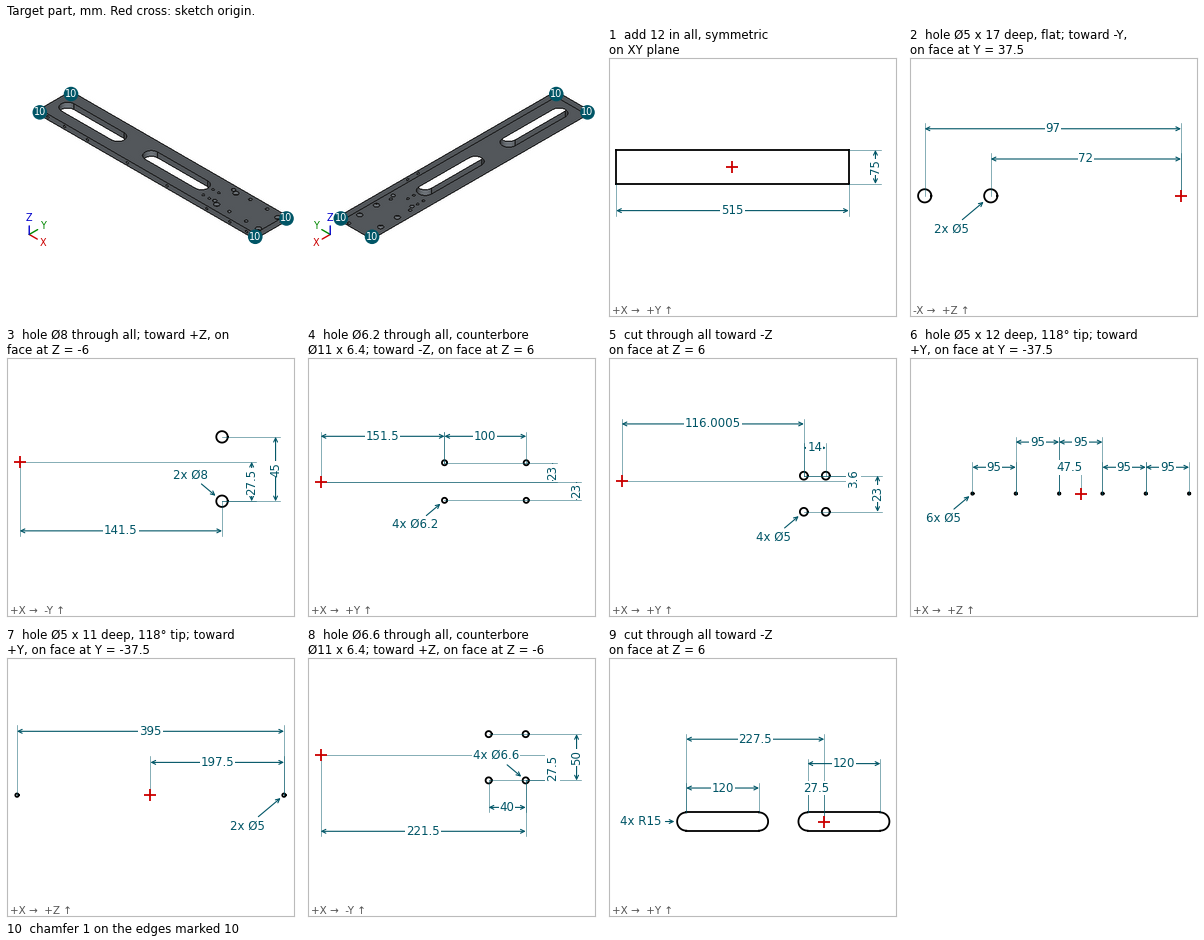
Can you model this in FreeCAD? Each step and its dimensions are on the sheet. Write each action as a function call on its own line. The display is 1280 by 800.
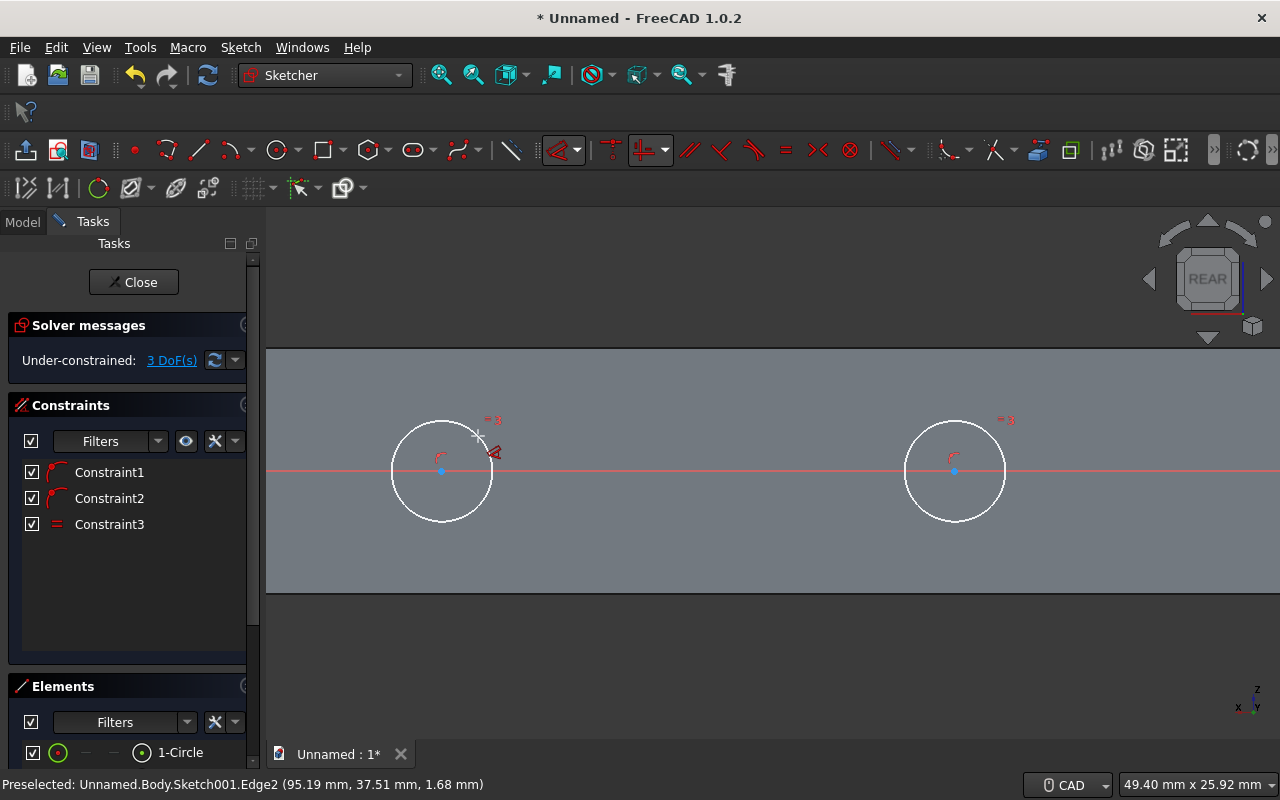
click(991, 436)
click(1014, 414)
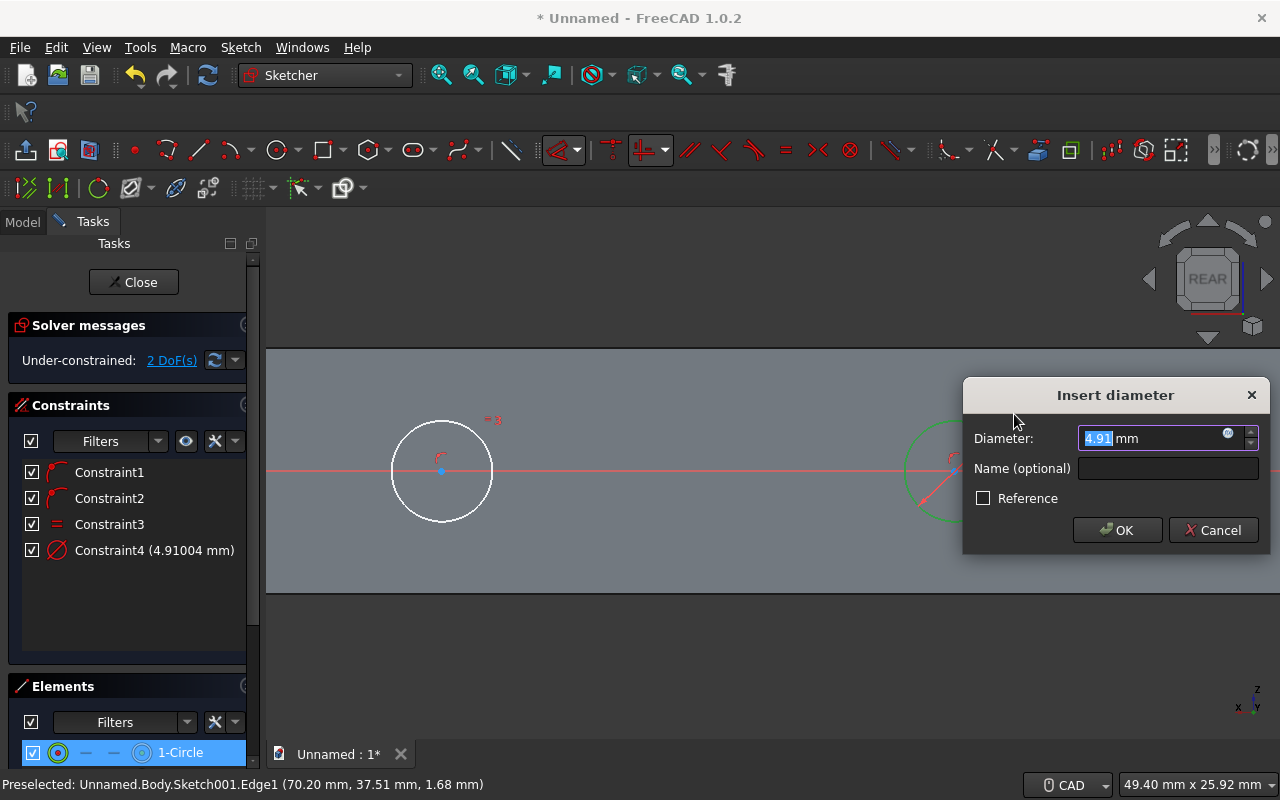
text(5)
key(Return)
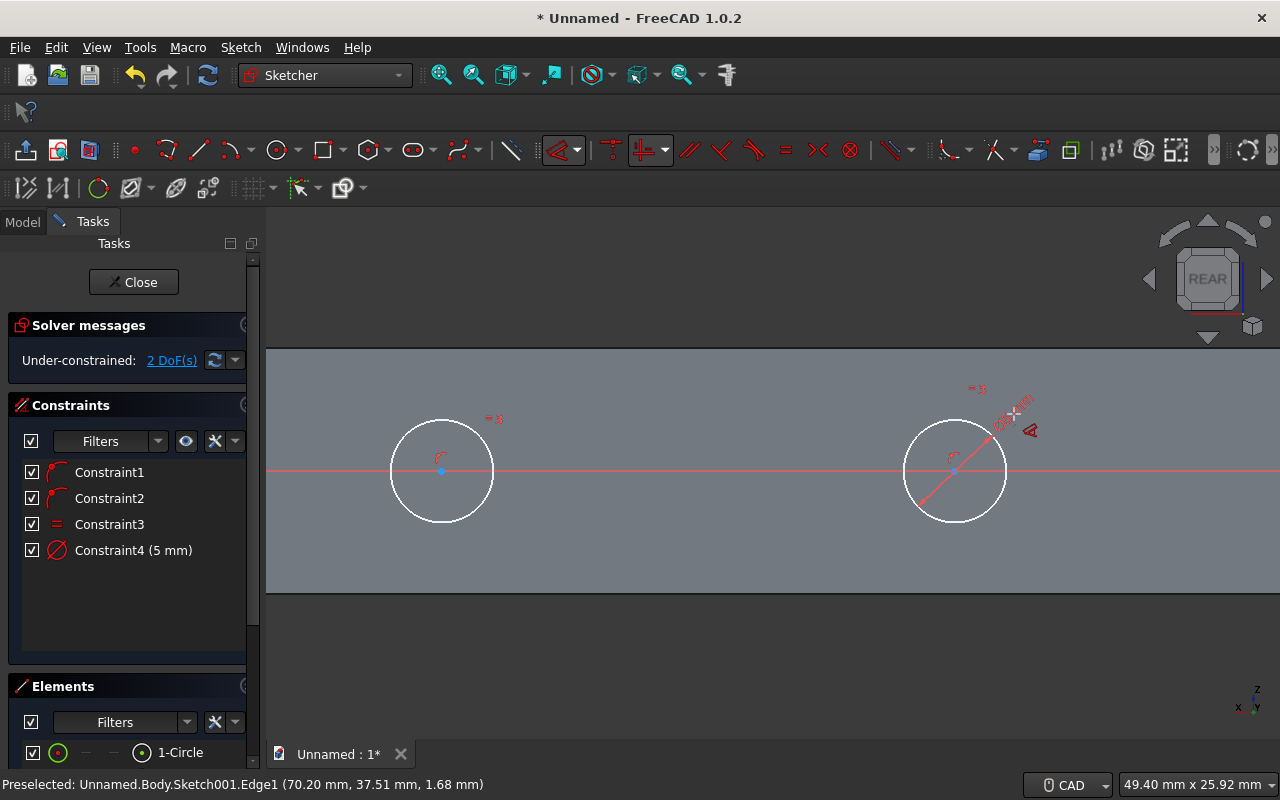
click(955, 471)
click(1035, 505)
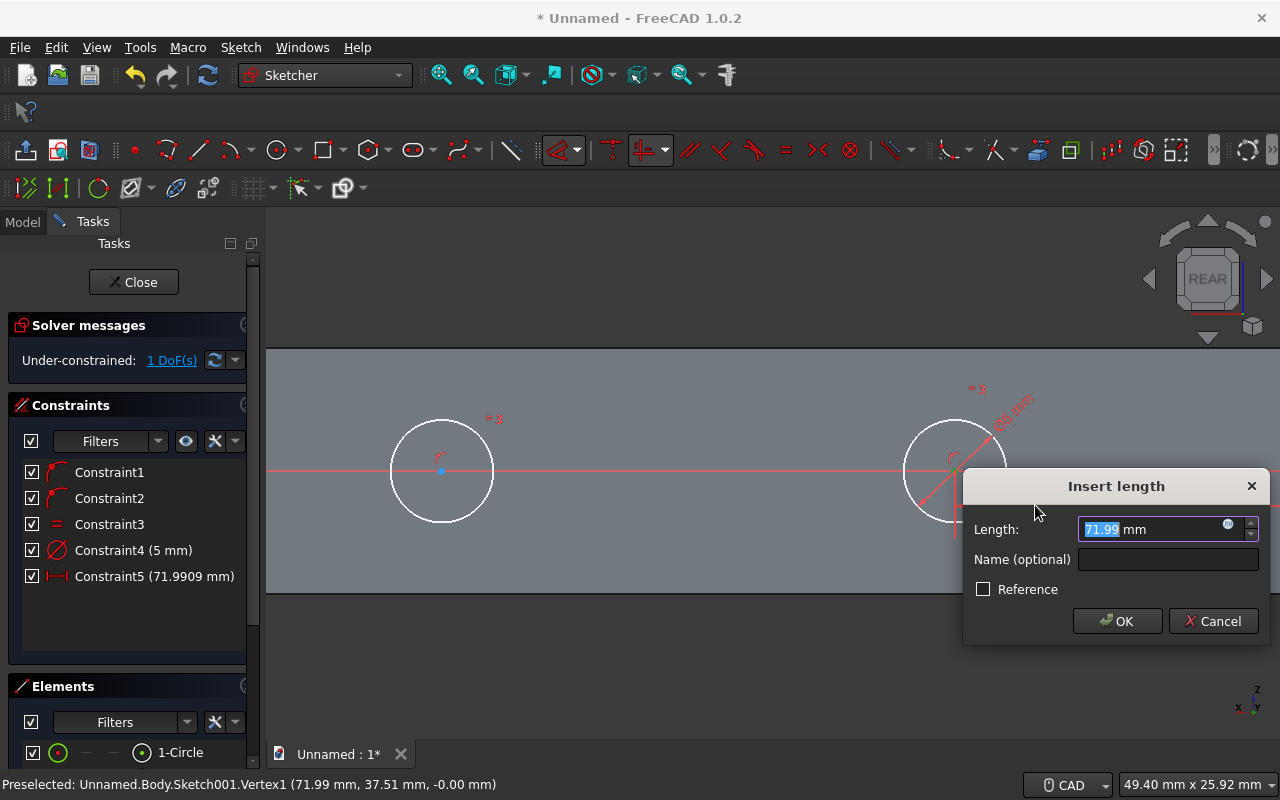
text(72)
key(Return)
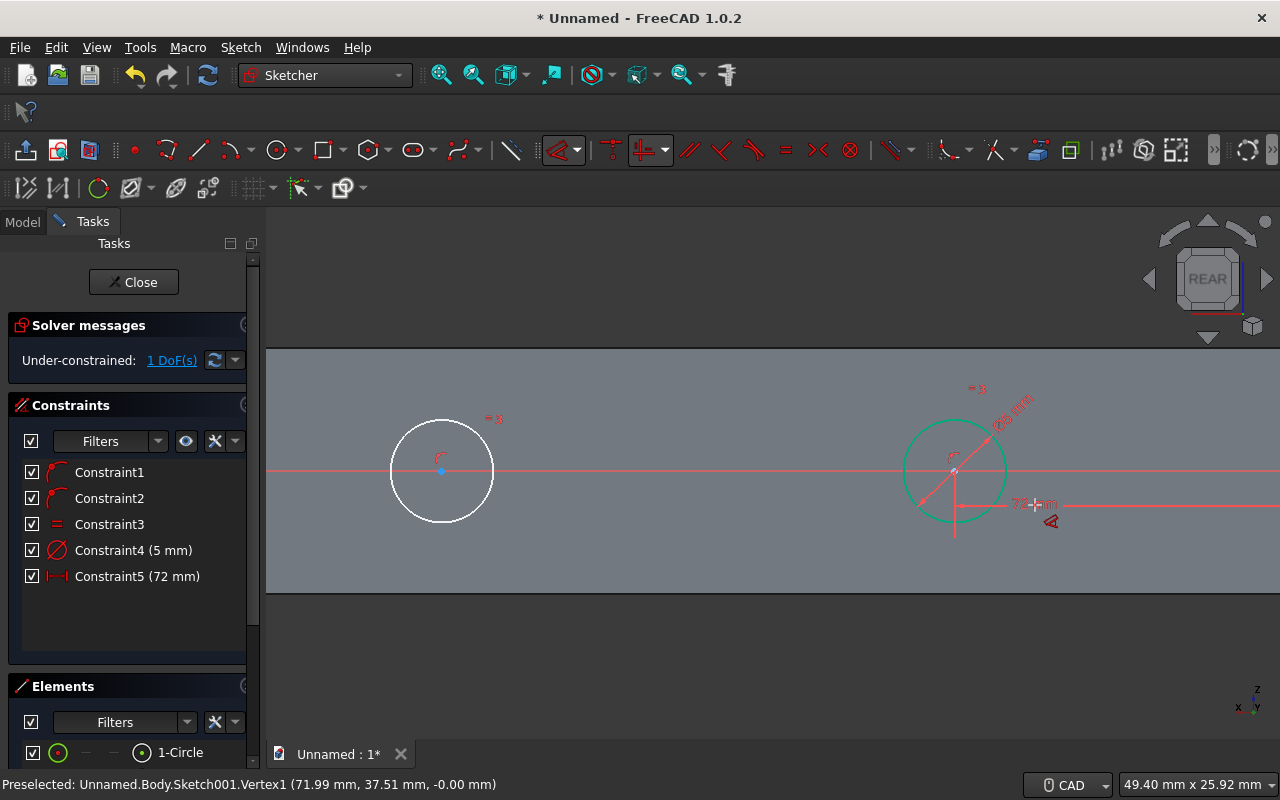
click(442, 471)
click(779, 505)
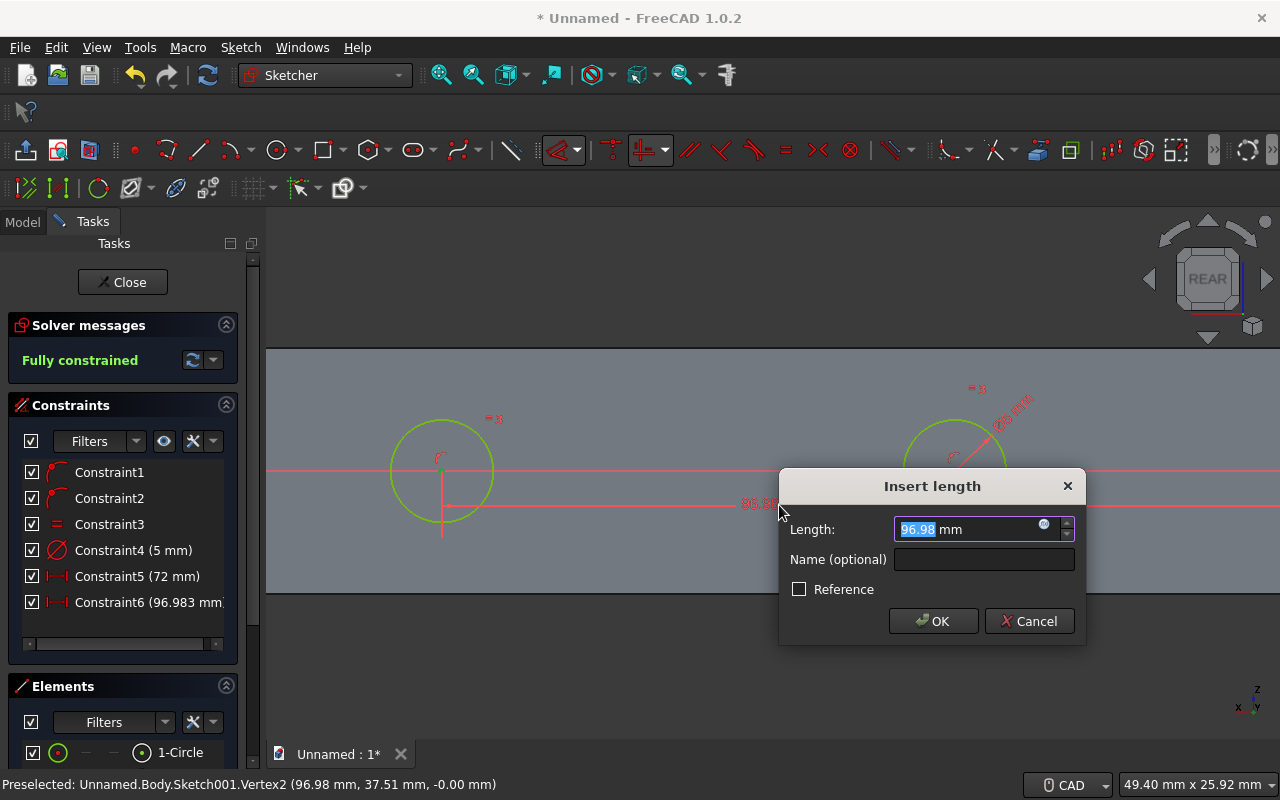
text(97)
key(Return)
key(Escape)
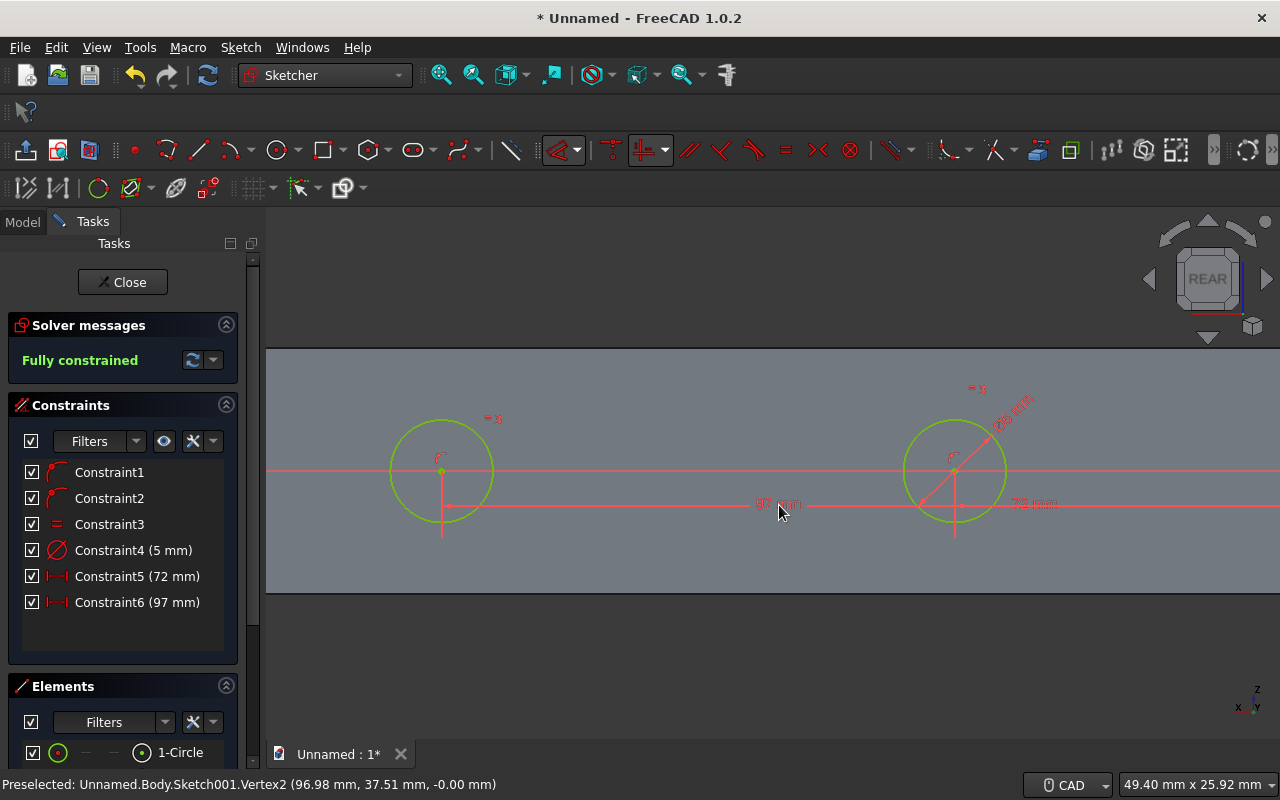
click(123, 282)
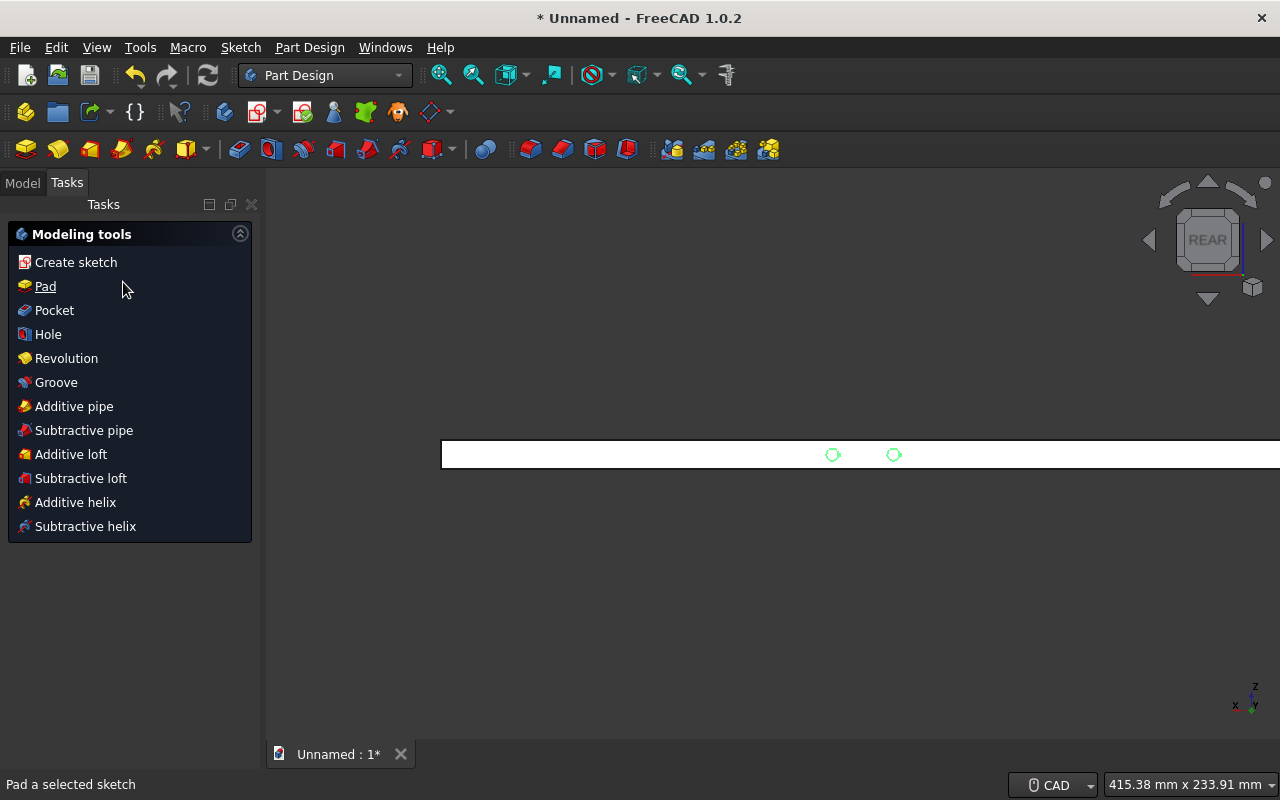
click(272, 150)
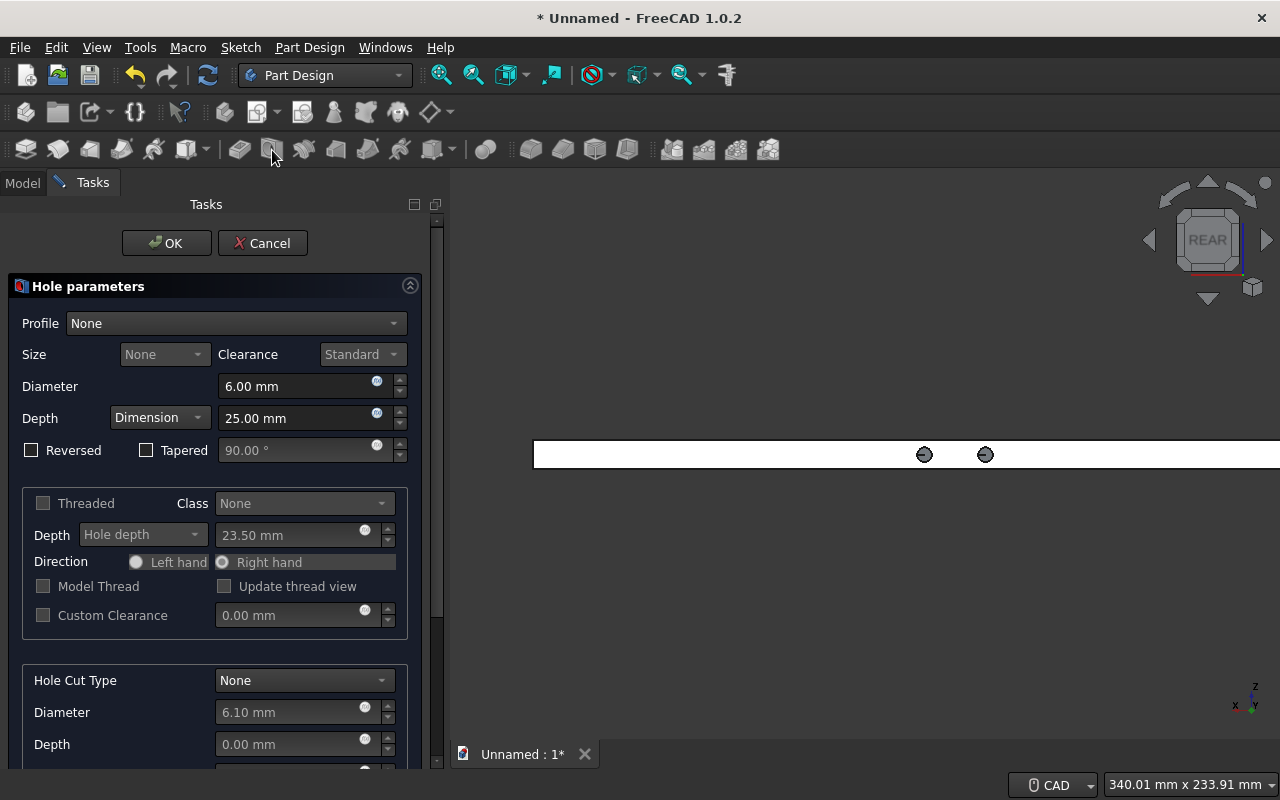
triple_click(305, 386)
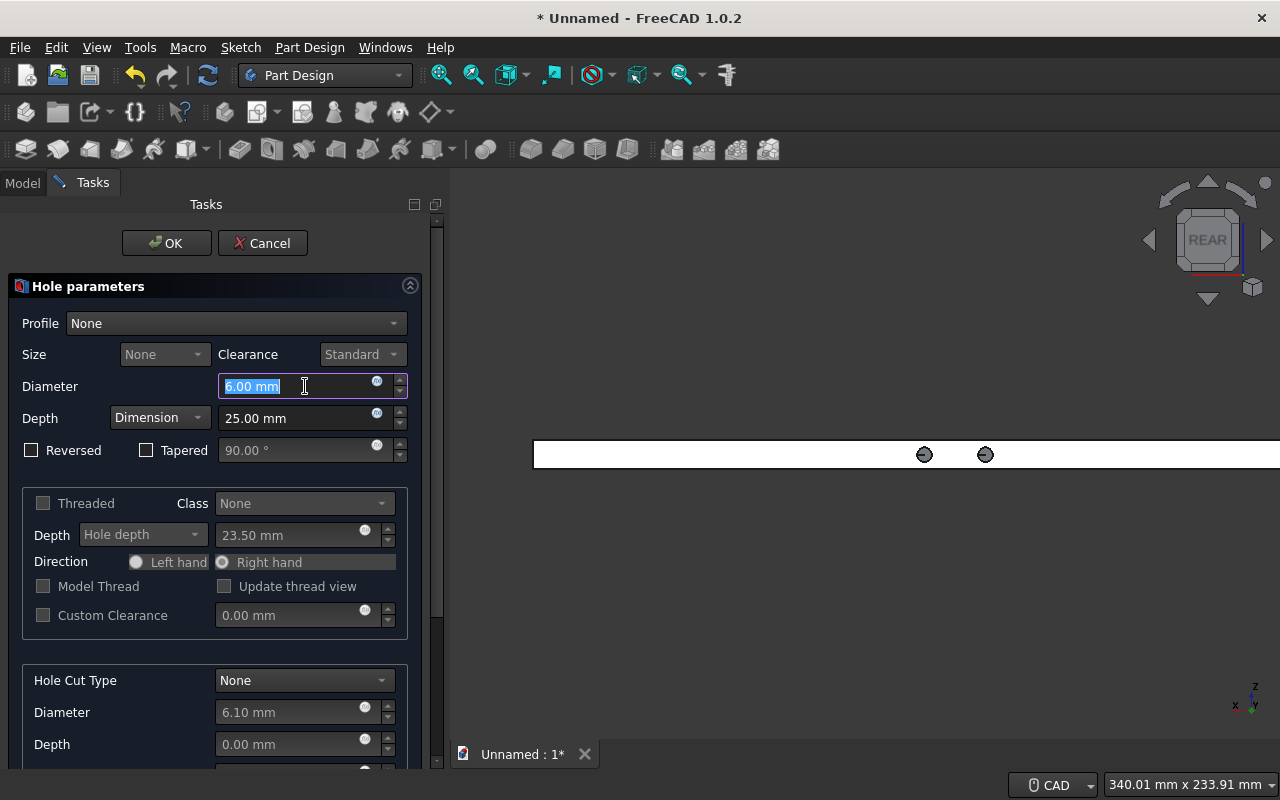
text(5)
key(Tab)